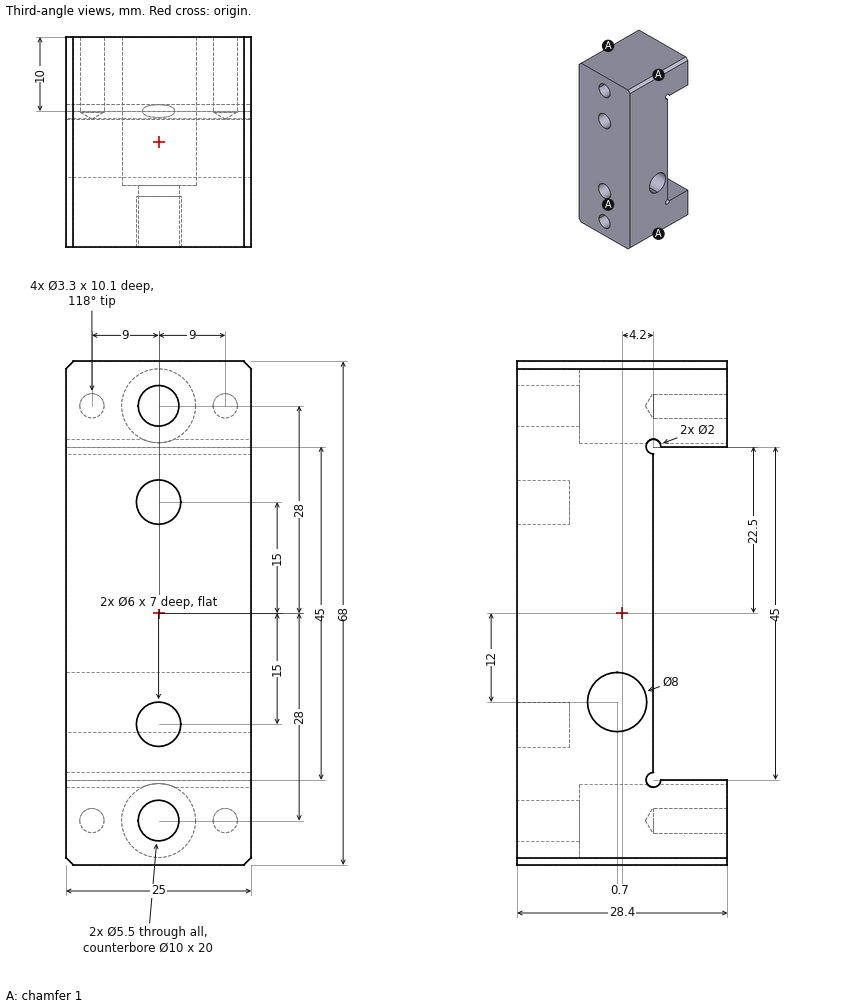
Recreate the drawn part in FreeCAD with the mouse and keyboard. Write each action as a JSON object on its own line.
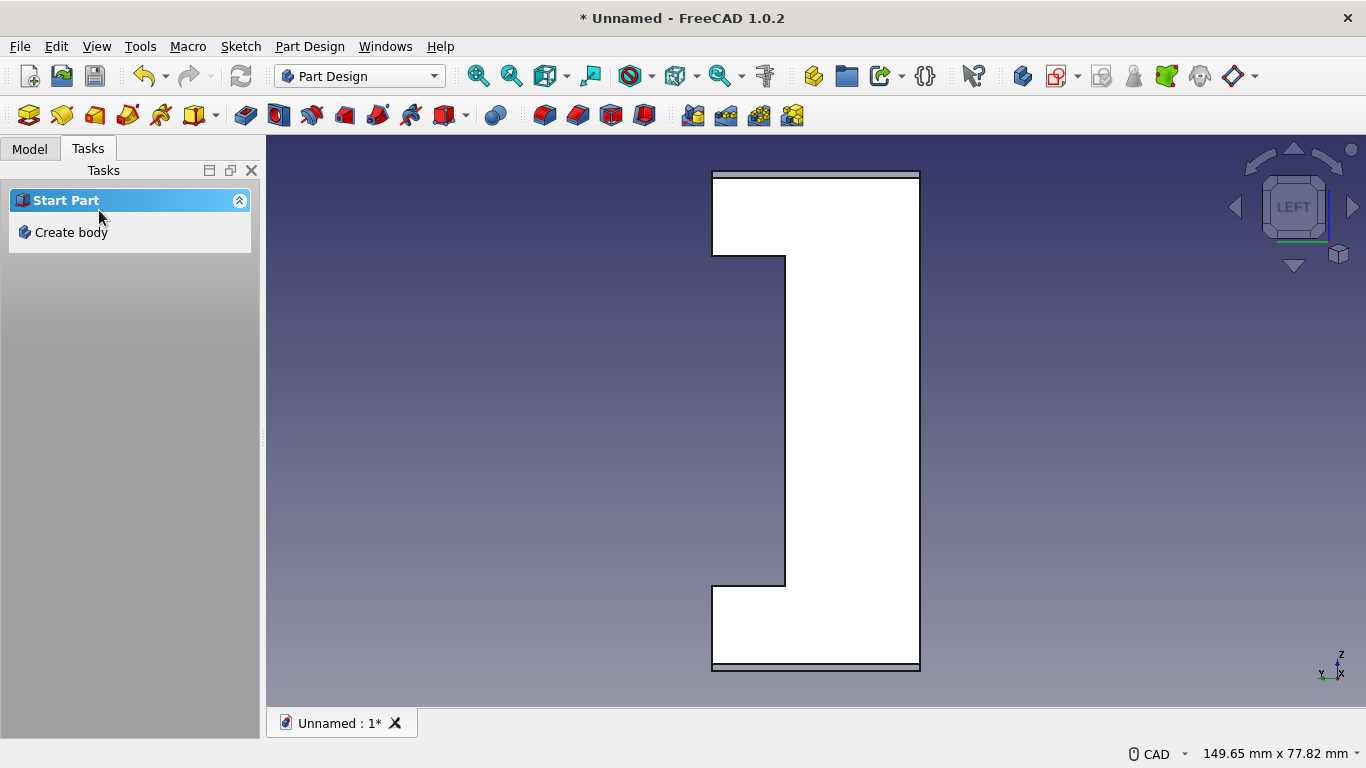
{"action": "left_click", "coordinate": [846, 559]}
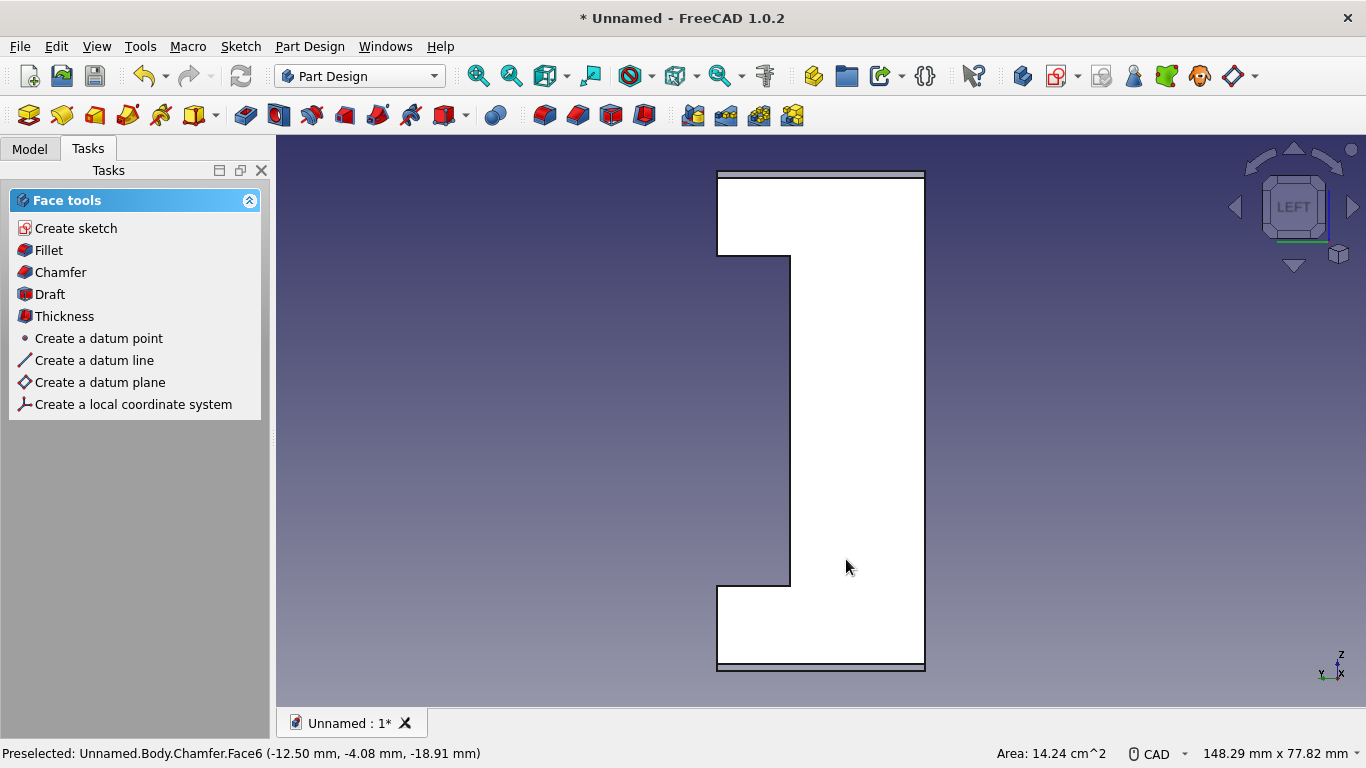
{"action": "left_click", "coordinate": [1056, 76]}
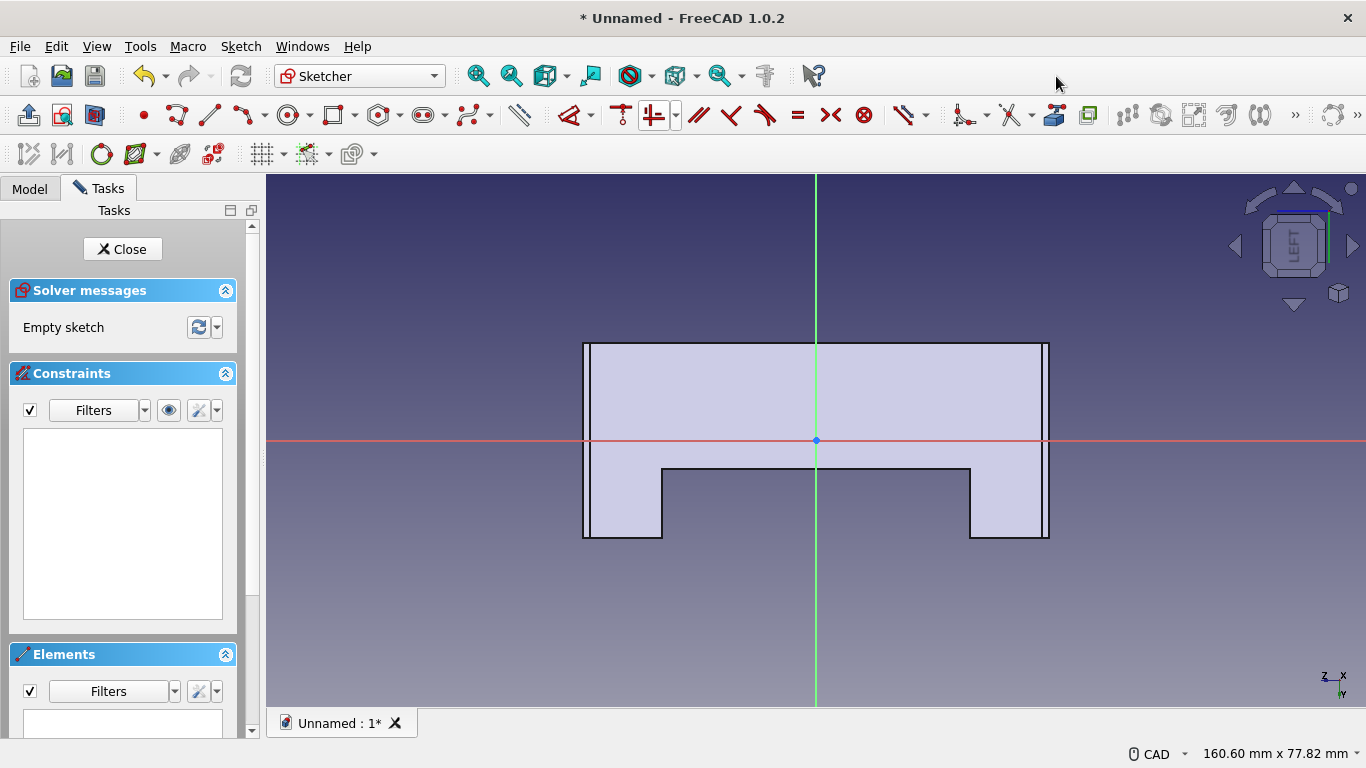
{"action": "scroll", "coordinate": [895, 435], "scroll_direction": "up", "scroll_amount": 9}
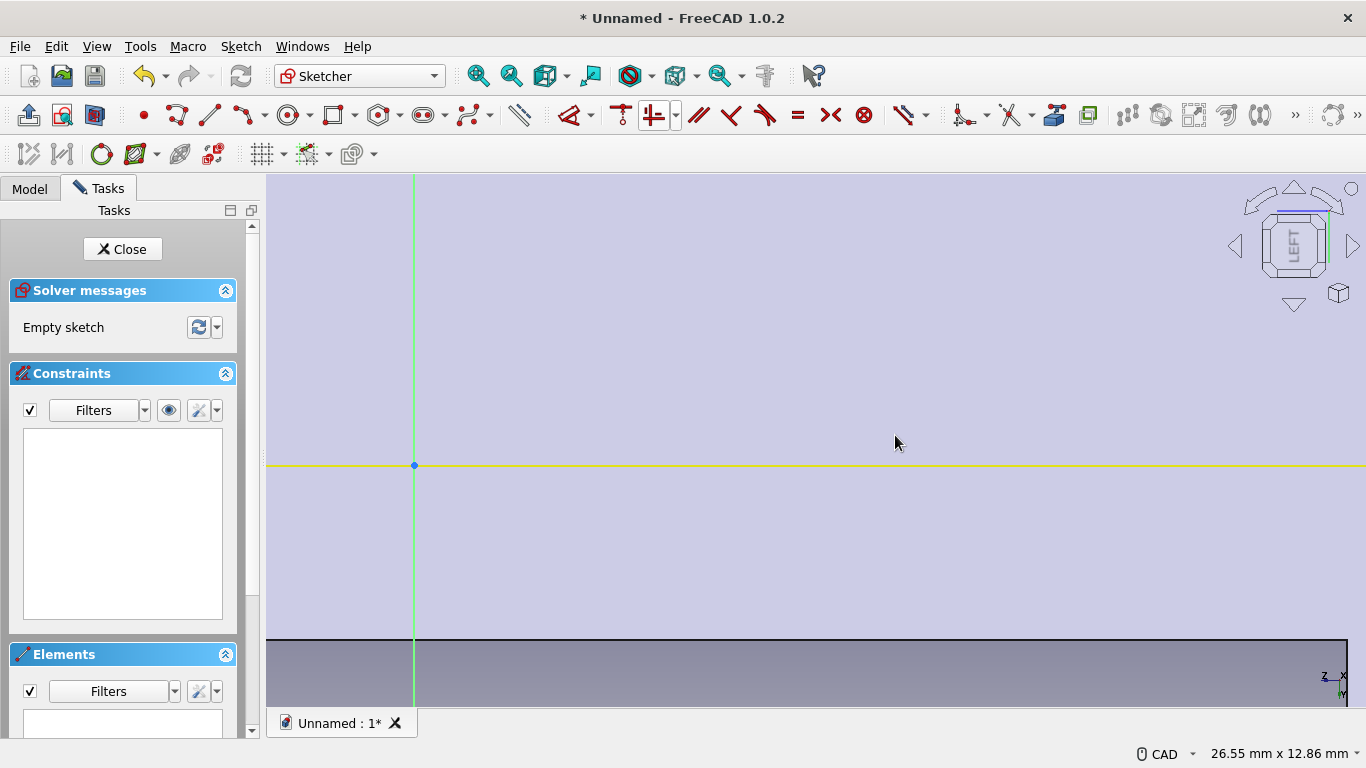
{"action": "key", "text": "g c"}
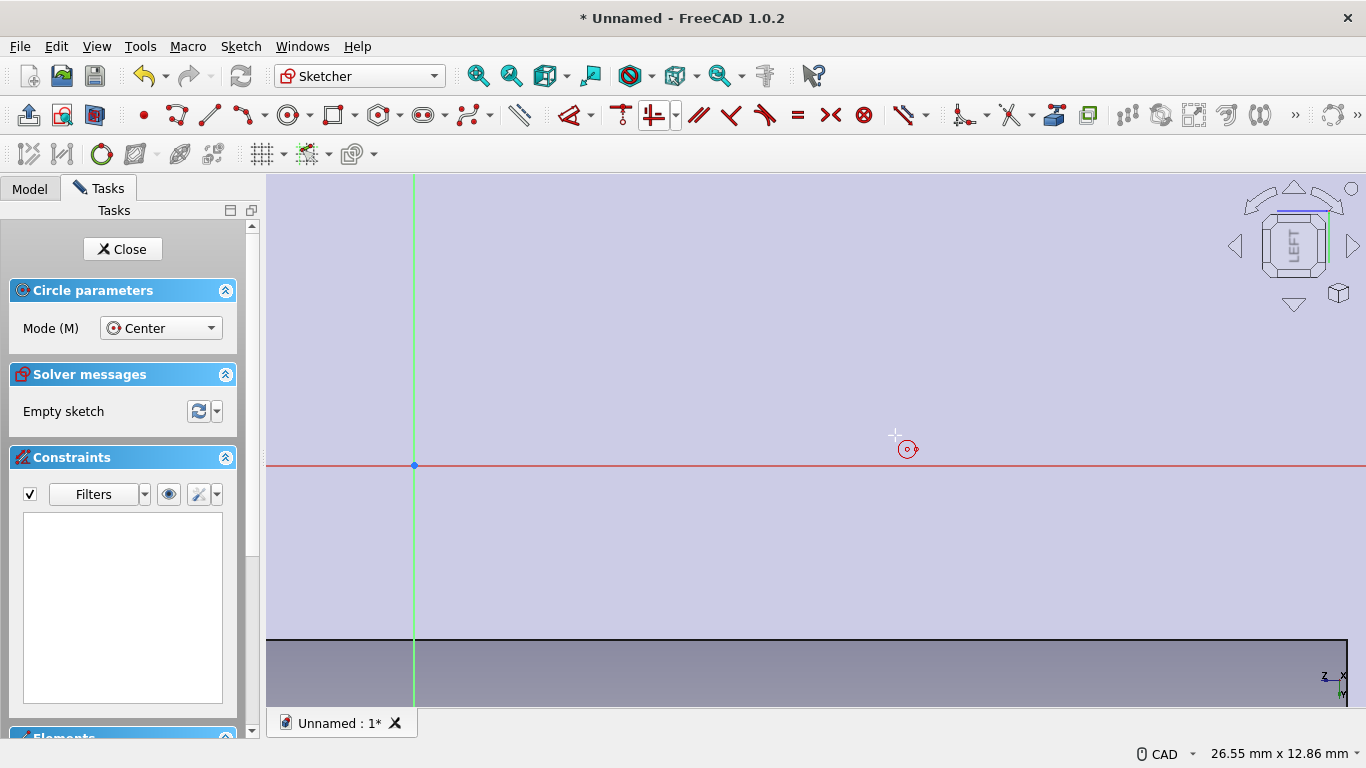
{"action": "left_click", "coordinate": [911, 437]}
{"action": "left_click", "coordinate": [1029, 320]}
{"action": "key", "text": "Escape"}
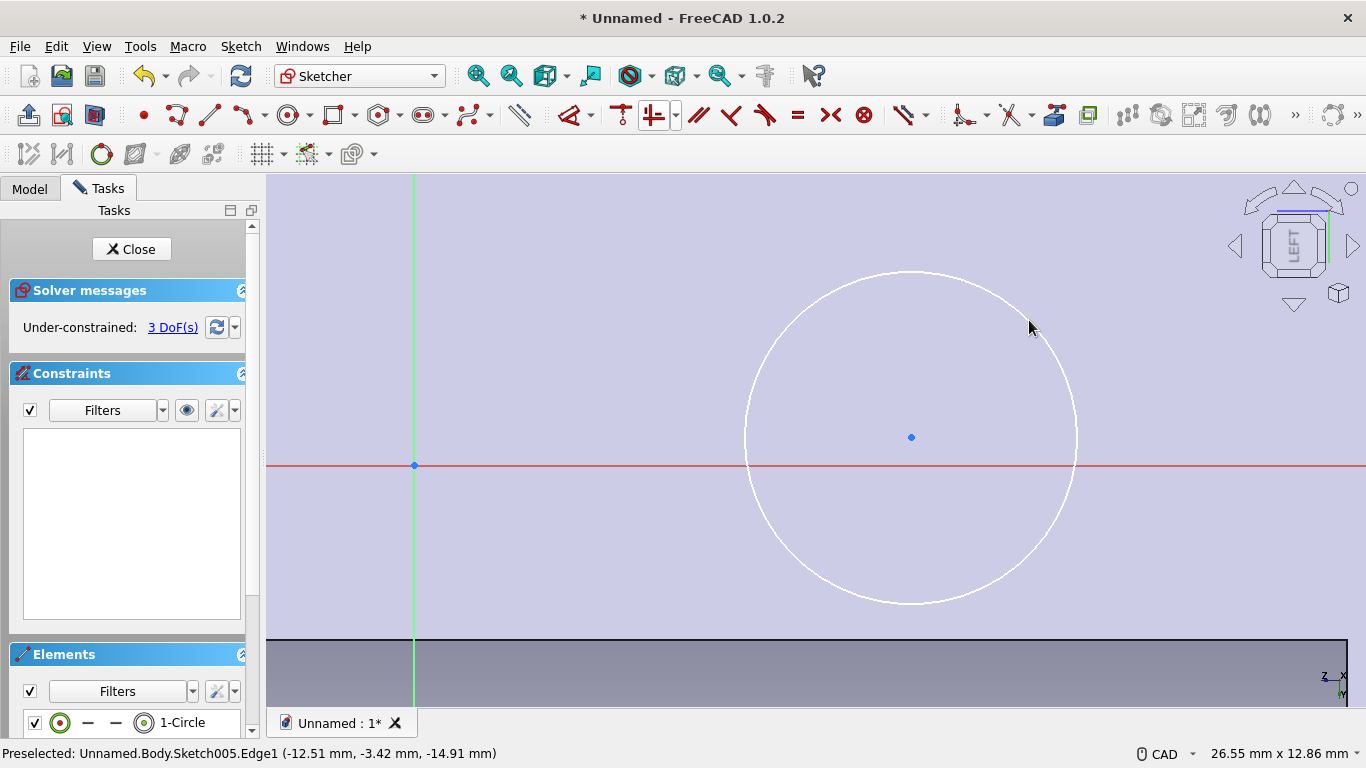
{"action": "left_click", "coordinate": [568, 116]}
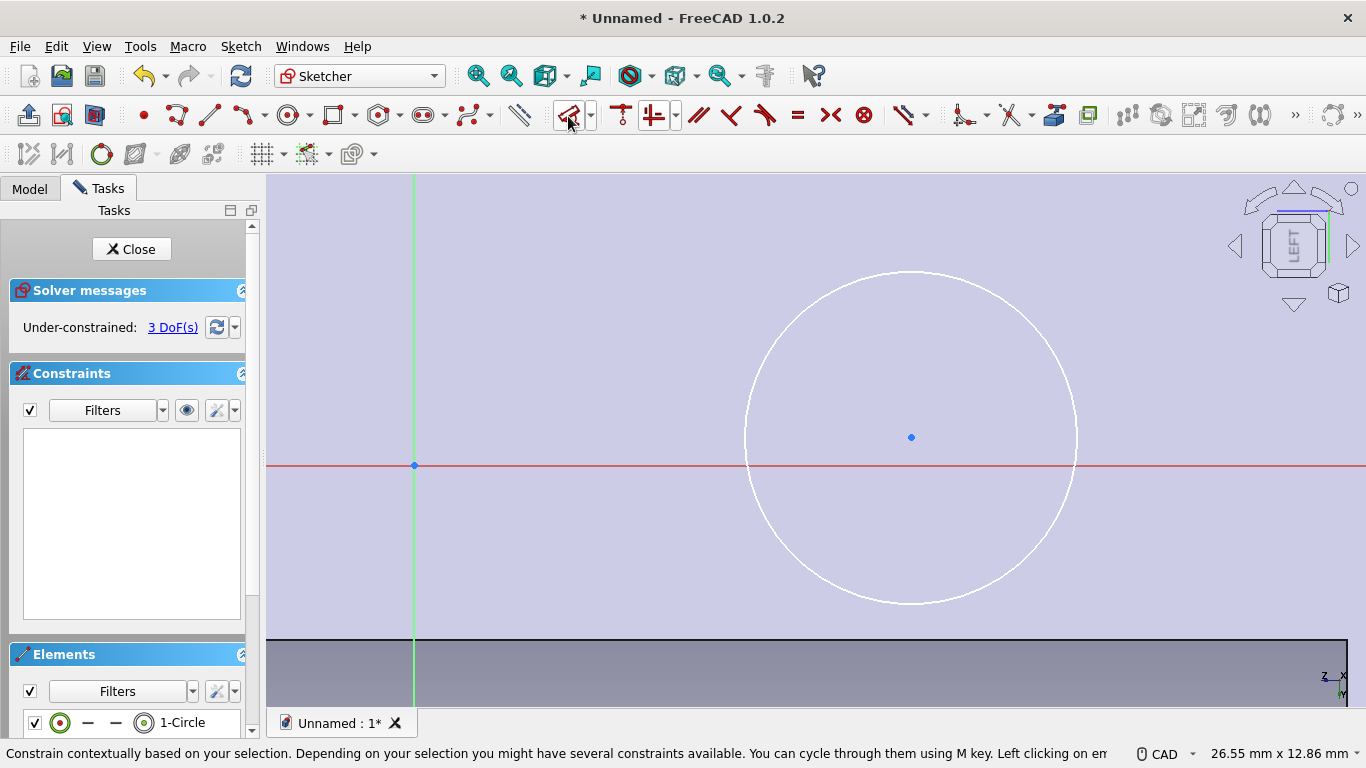
{"action": "left_click", "coordinate": [1028, 320]}
{"action": "left_click", "coordinate": [1051, 297]}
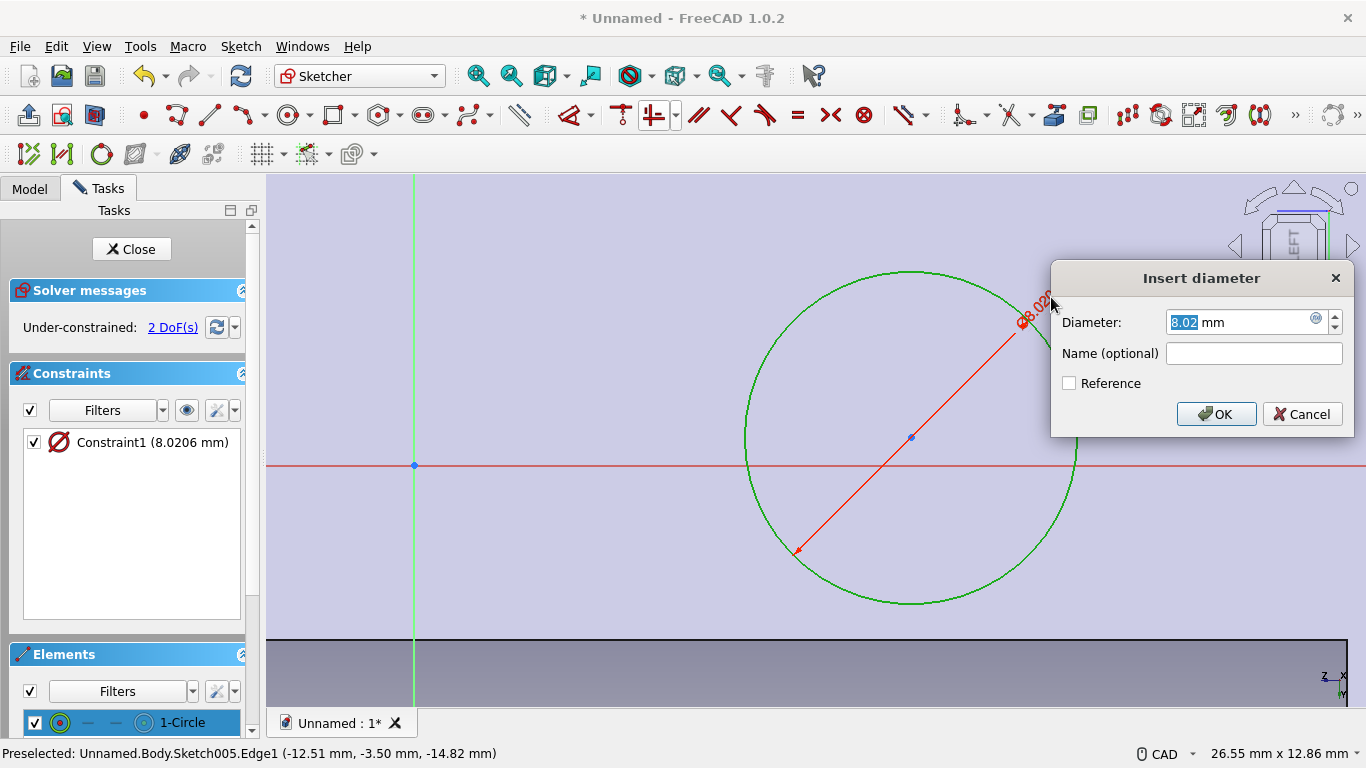
{"action": "type", "text": "8"}
{"action": "key", "text": "Return"}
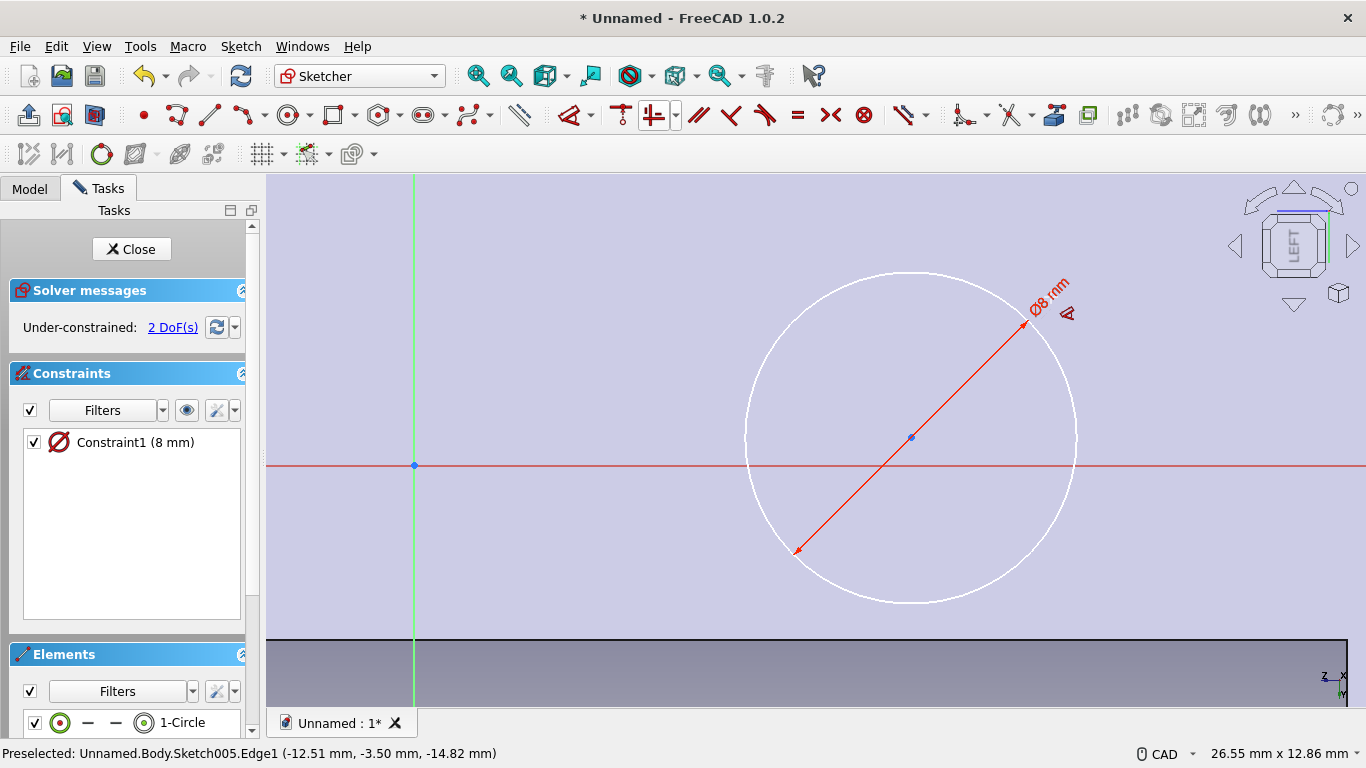
{"action": "left_click", "coordinate": [911, 438]}
{"action": "left_click", "coordinate": [663, 500]}